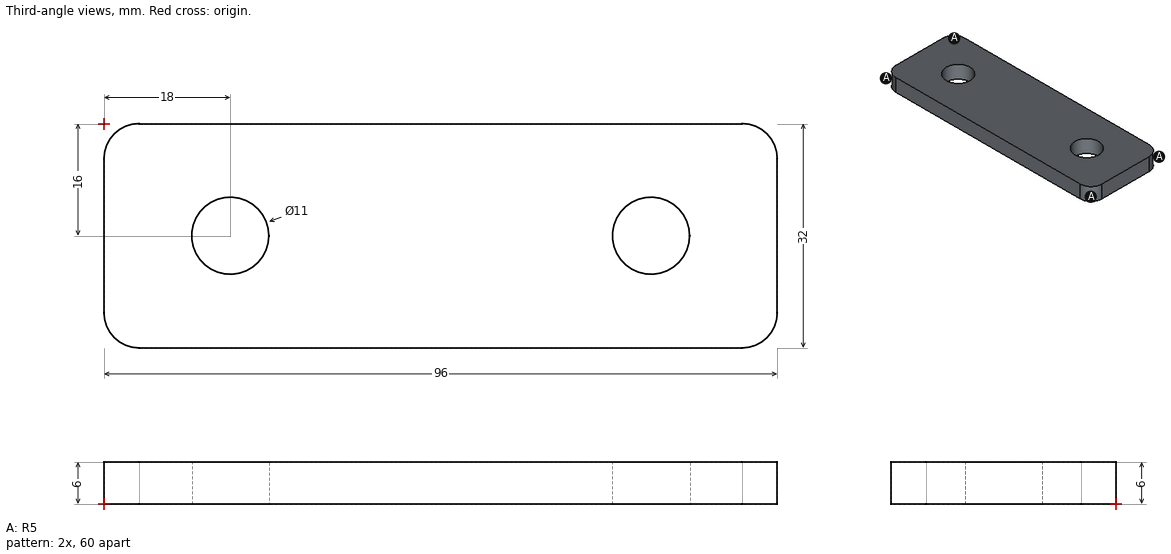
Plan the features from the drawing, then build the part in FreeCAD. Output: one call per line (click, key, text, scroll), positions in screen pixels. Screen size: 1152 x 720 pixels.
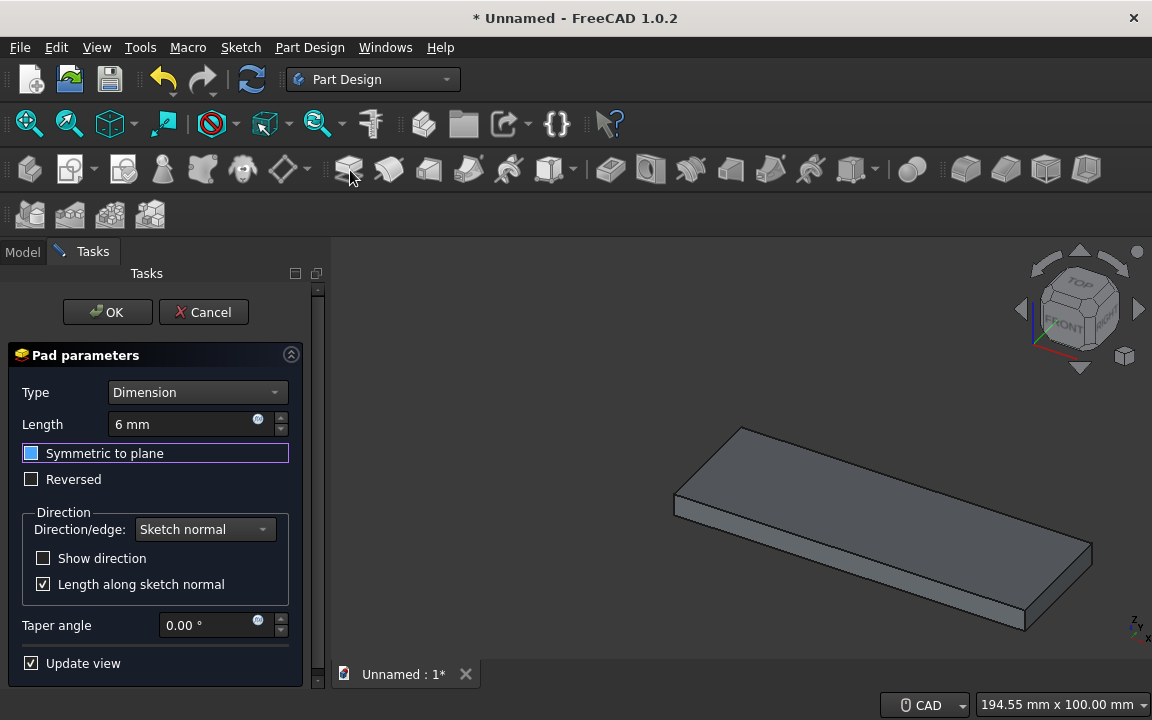
click(108, 312)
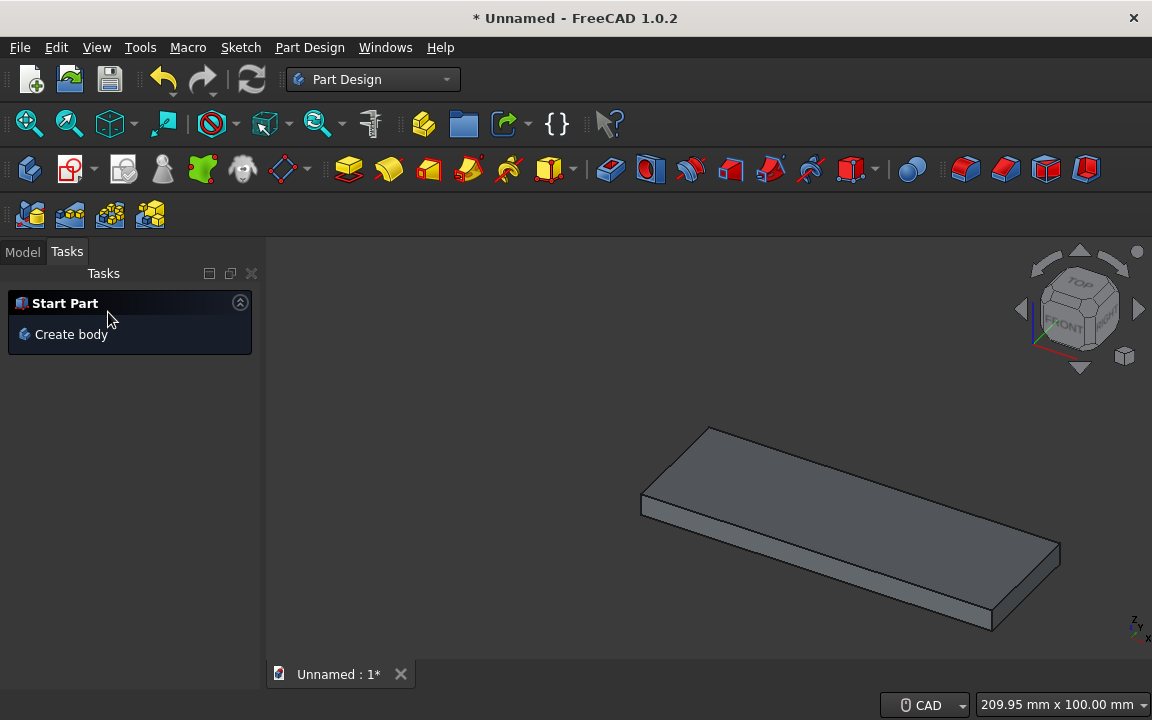
click(992, 620)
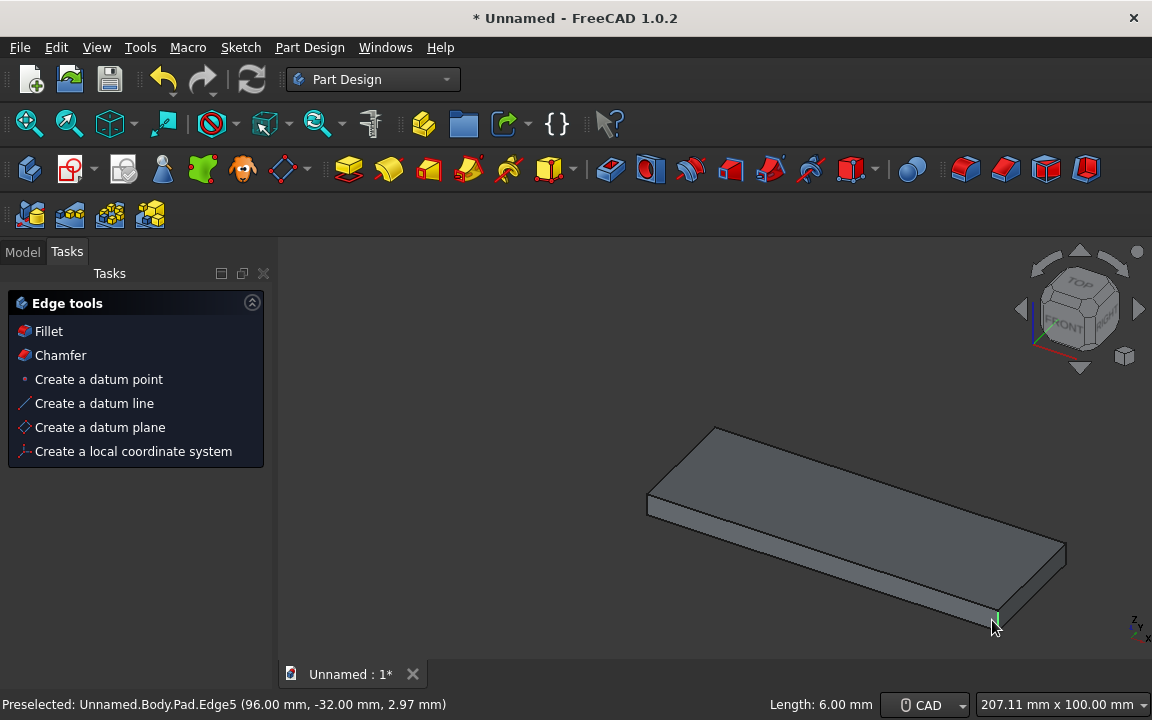
key(0)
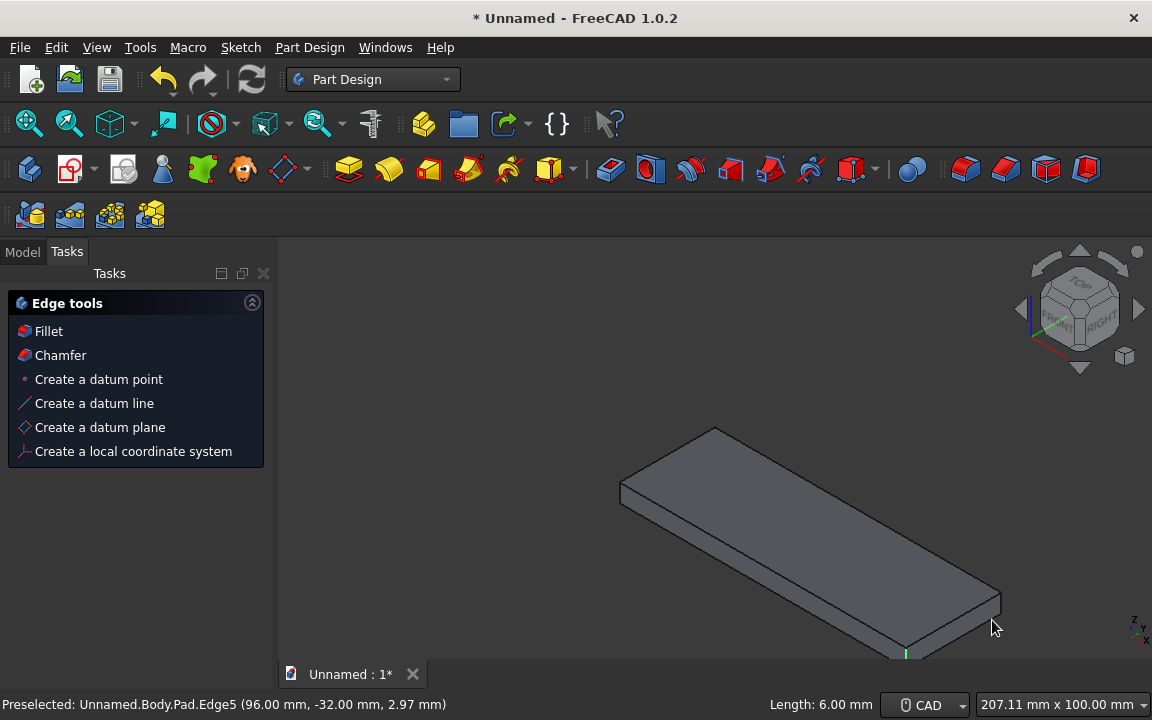
click(30, 124)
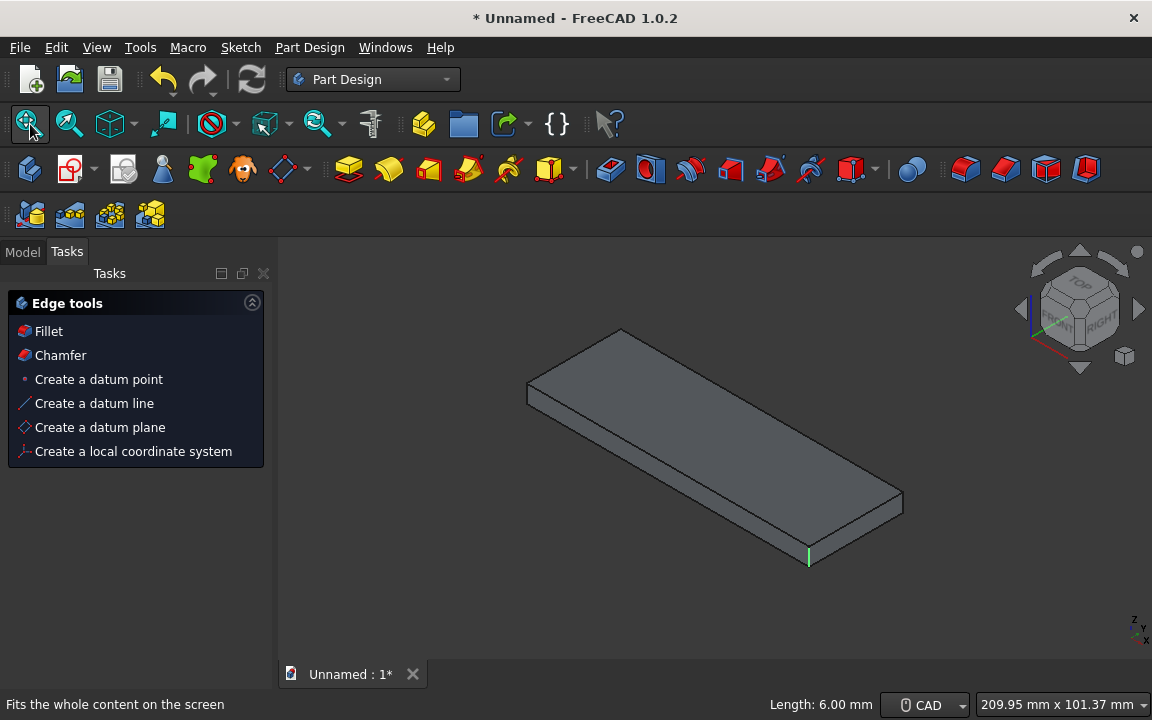
key(2)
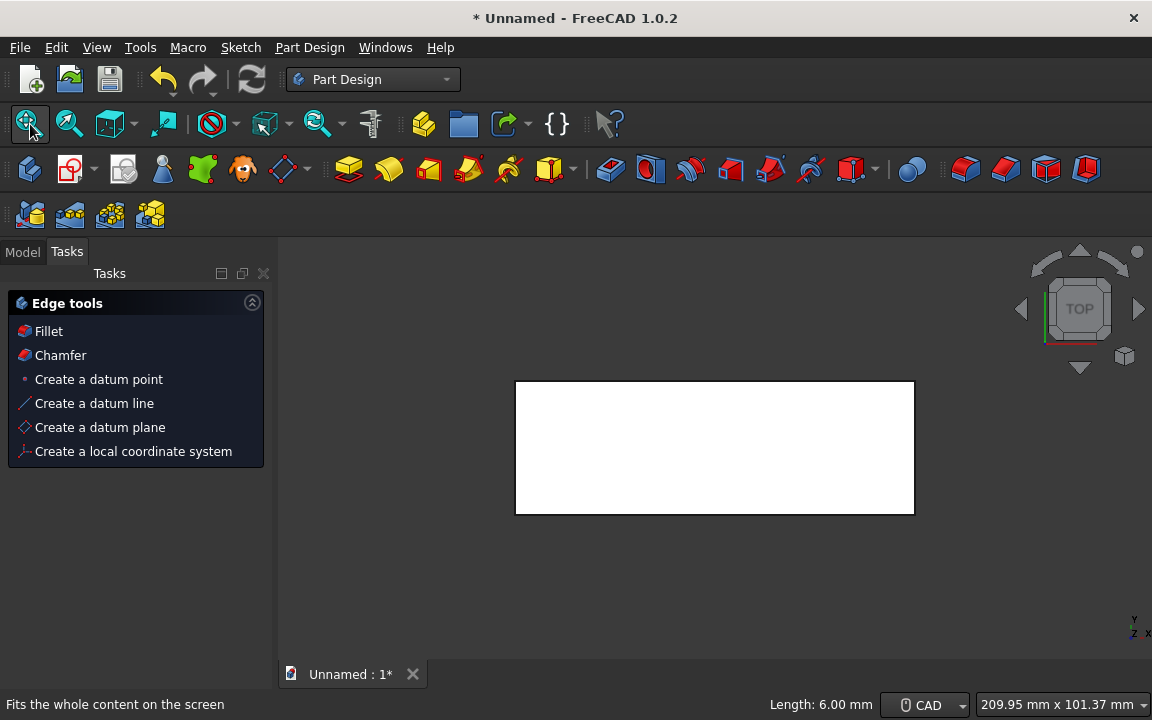
key(1)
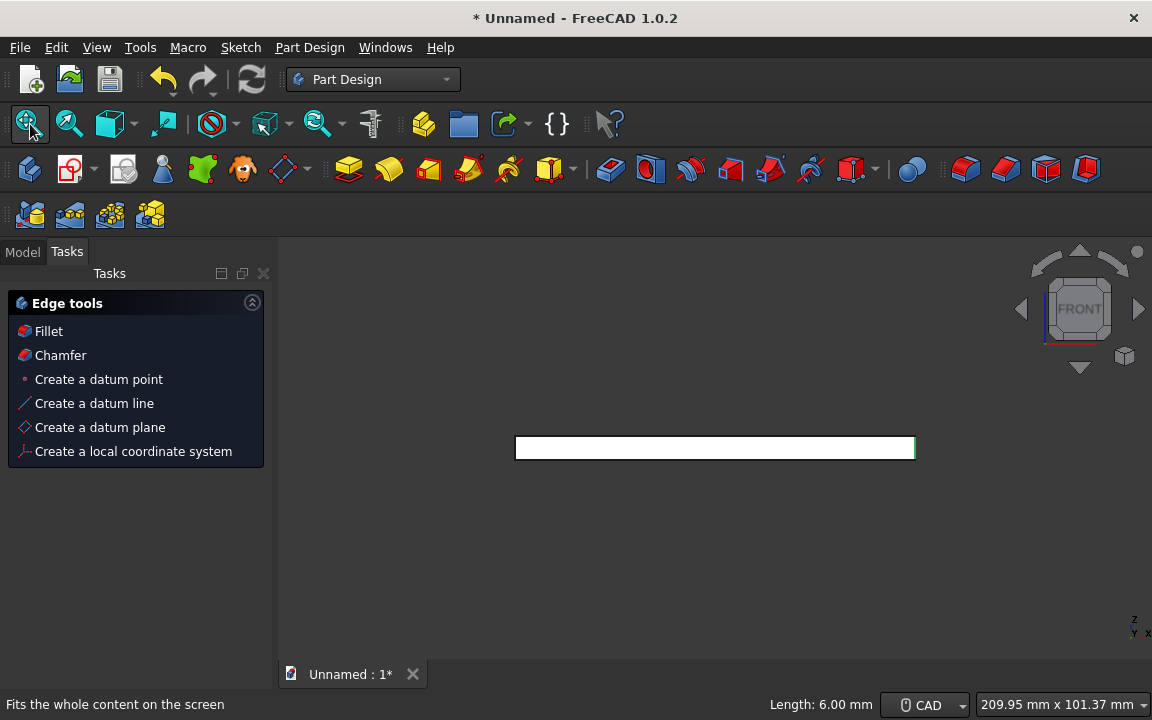
click(515, 447, ctrl)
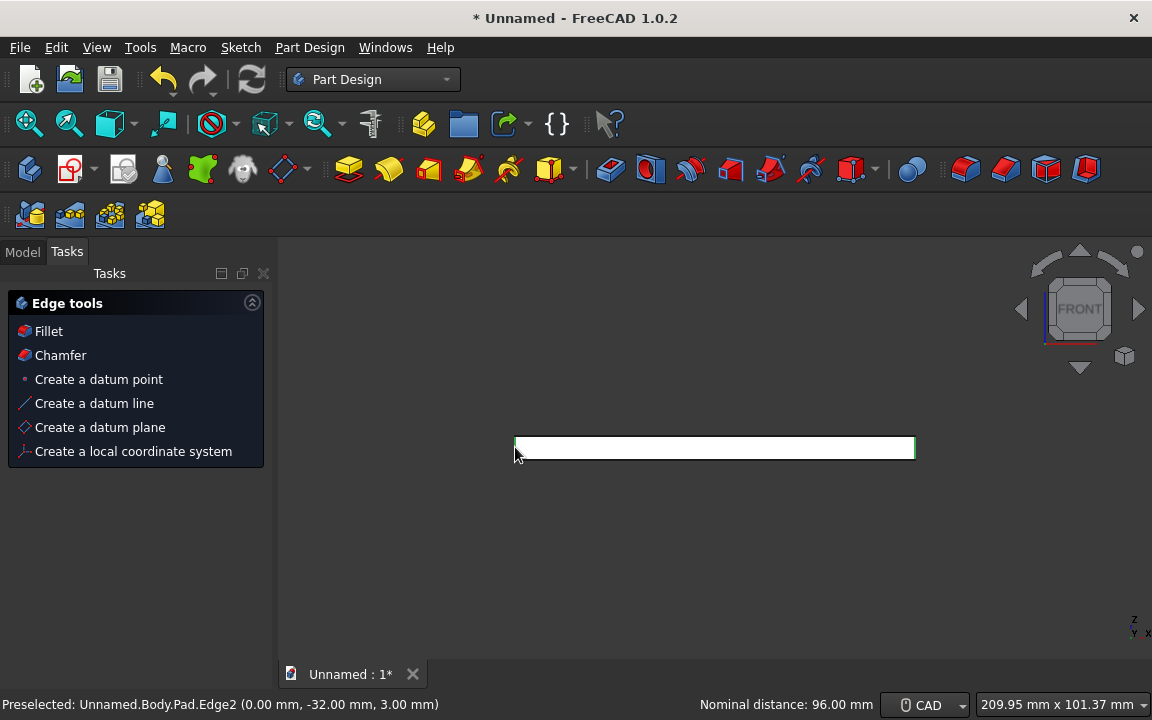
key(3)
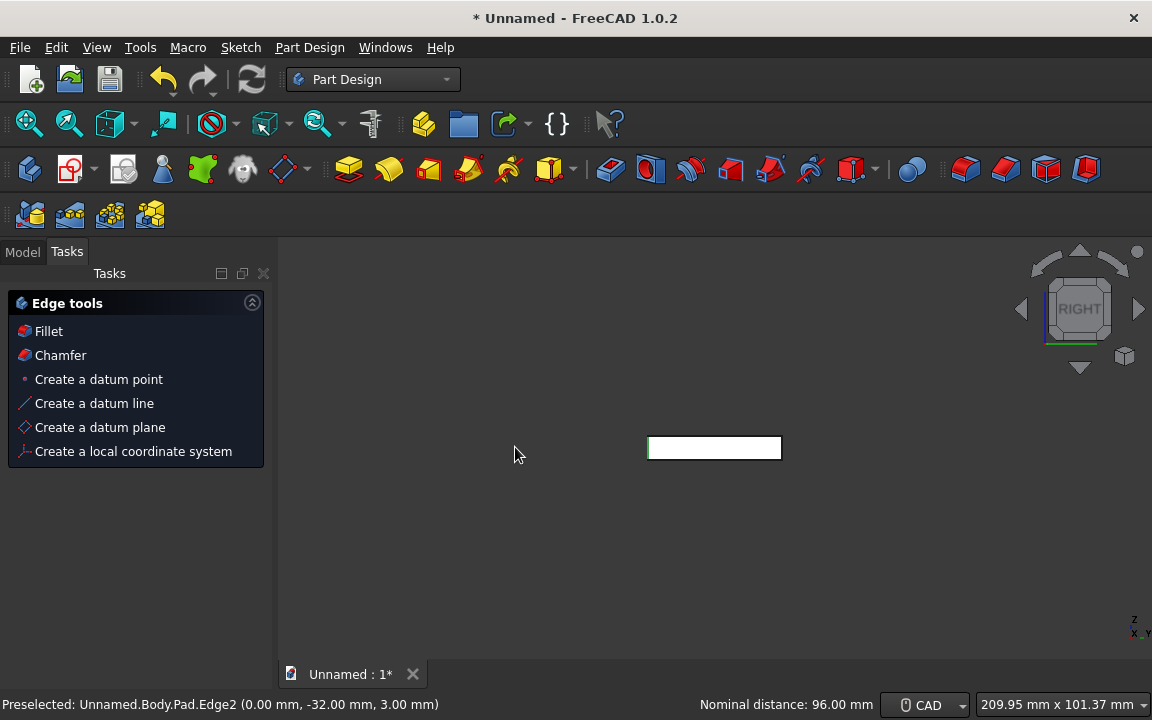
key(v)
key(f)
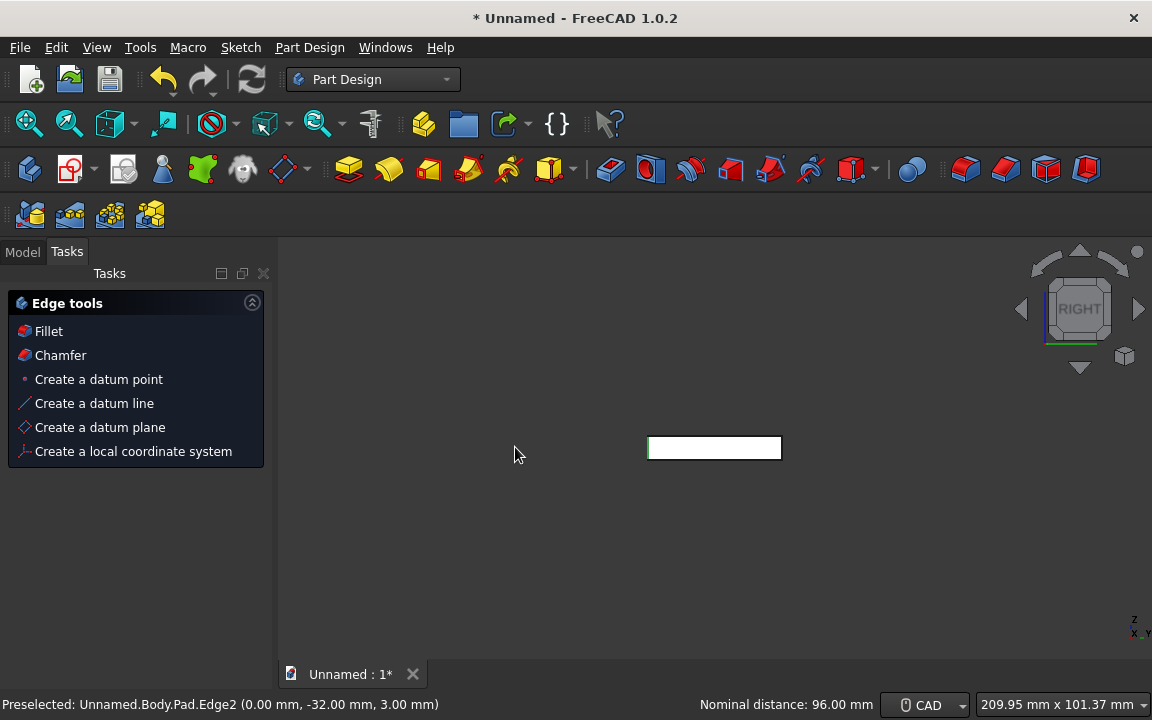
click(782, 447, ctrl)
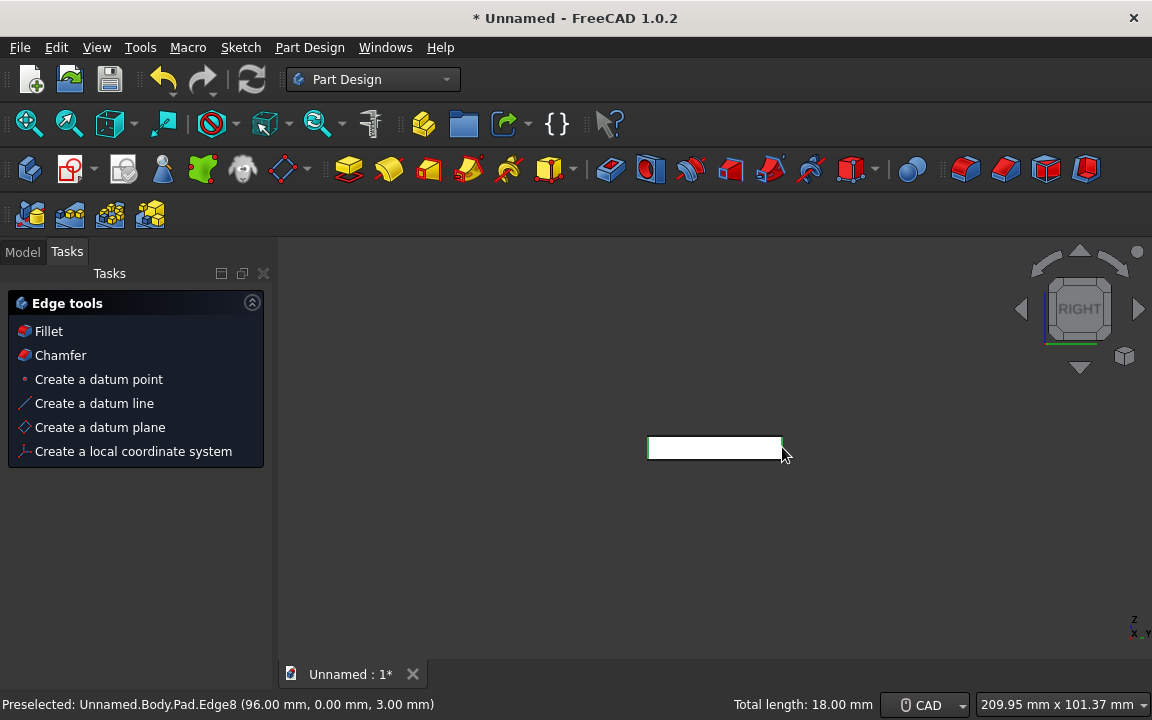
key(5)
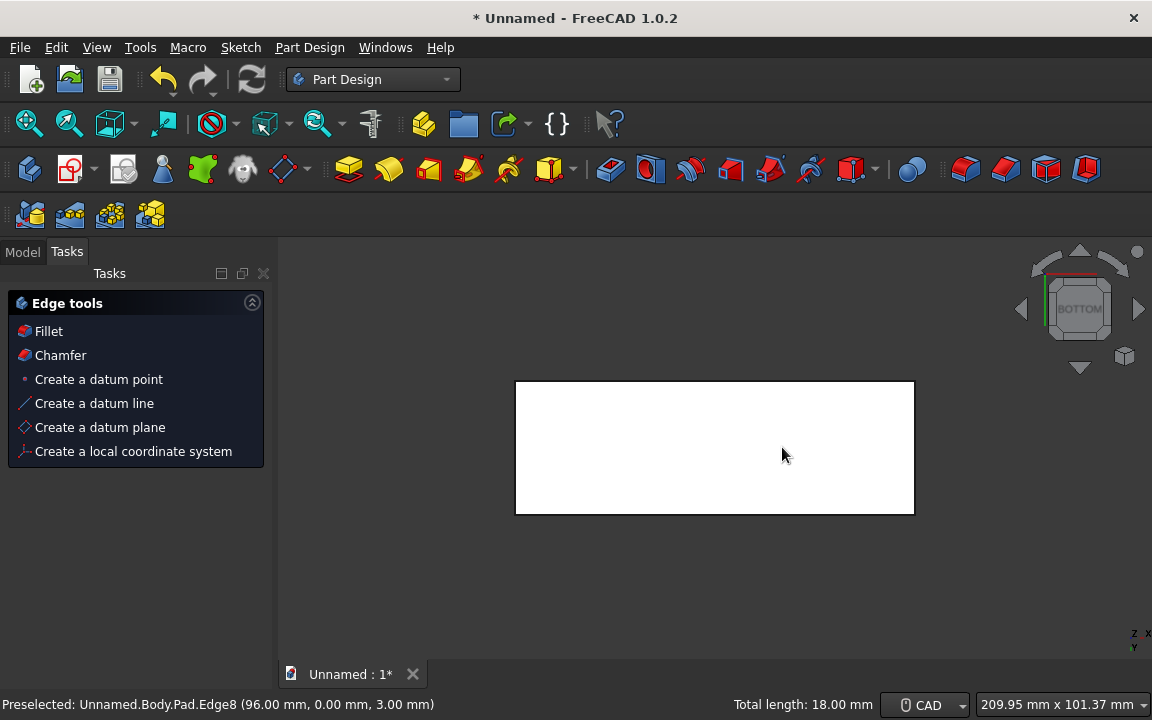
key(4)